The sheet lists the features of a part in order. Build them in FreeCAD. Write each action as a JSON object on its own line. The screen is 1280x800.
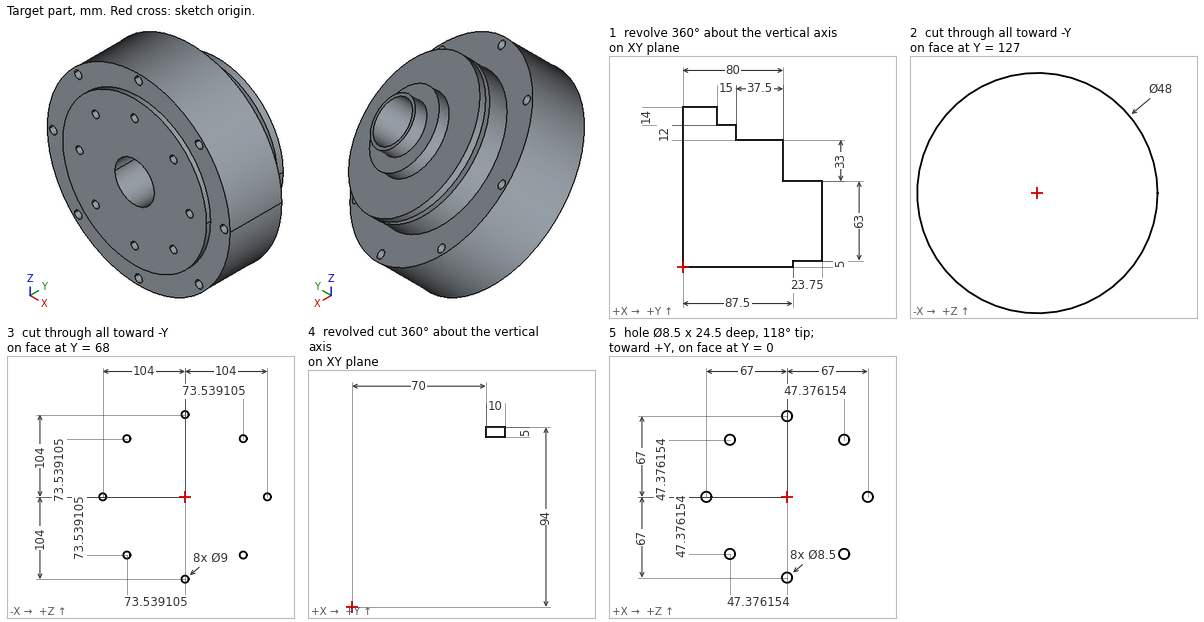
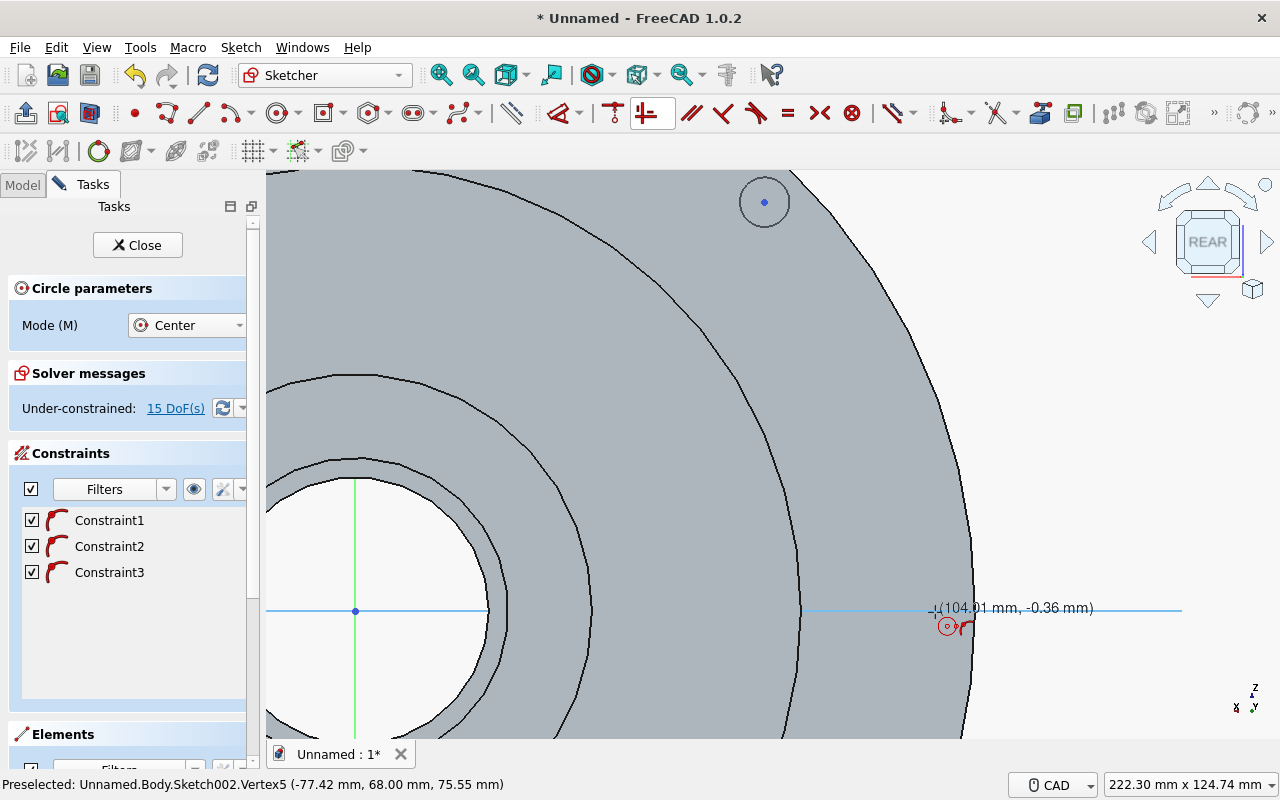
{"action": "left_click", "coordinate": [935, 611]}
{"action": "left_click", "coordinate": [952, 593]}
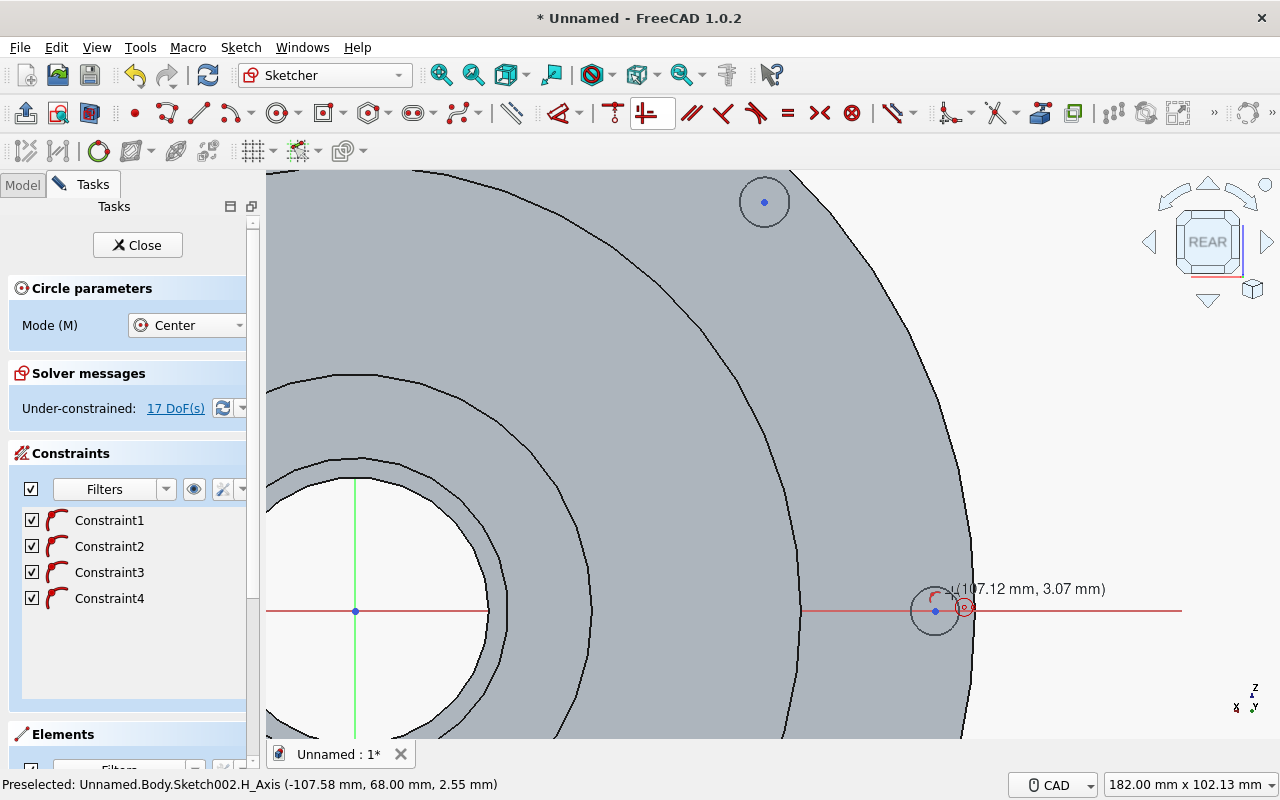
{"action": "scroll", "coordinate": [855, 387], "scroll_direction": "down", "scroll_amount": 6}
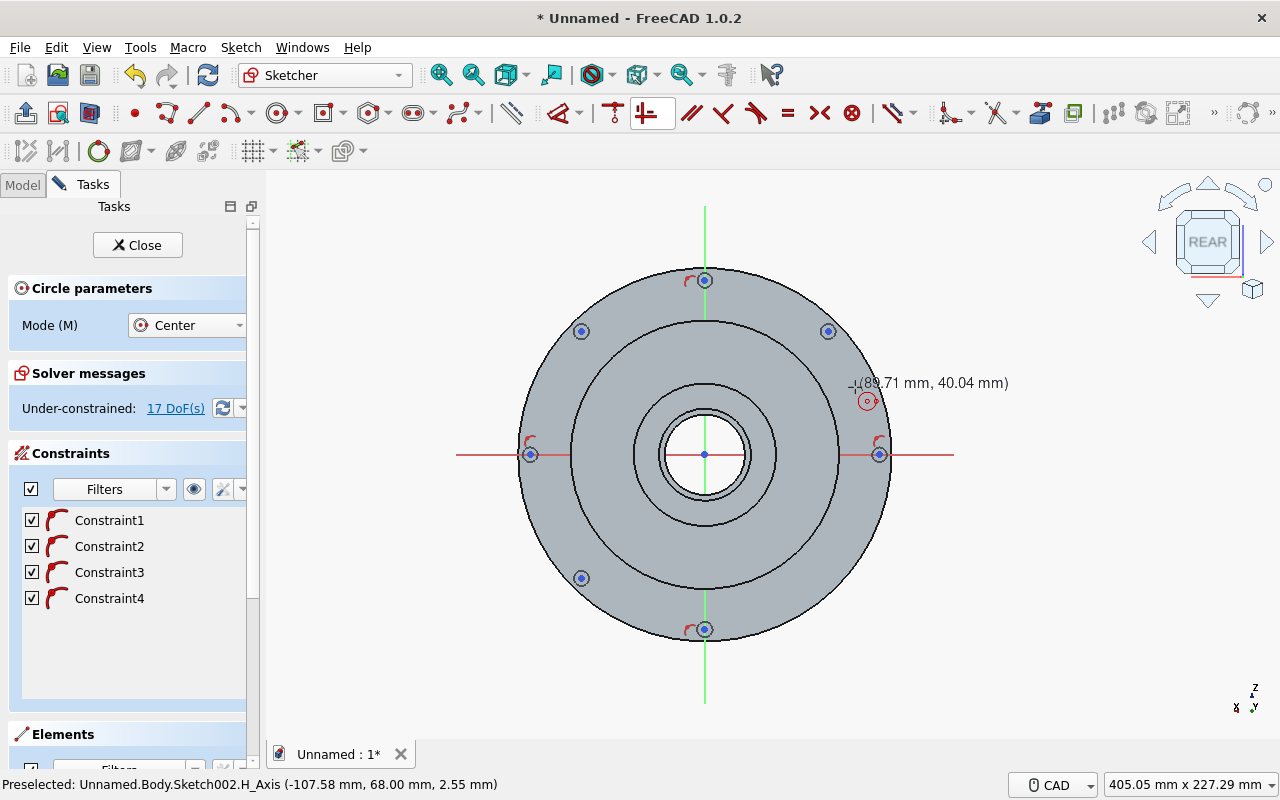
{"action": "scroll", "coordinate": [828, 578], "scroll_direction": "up", "scroll_amount": 6}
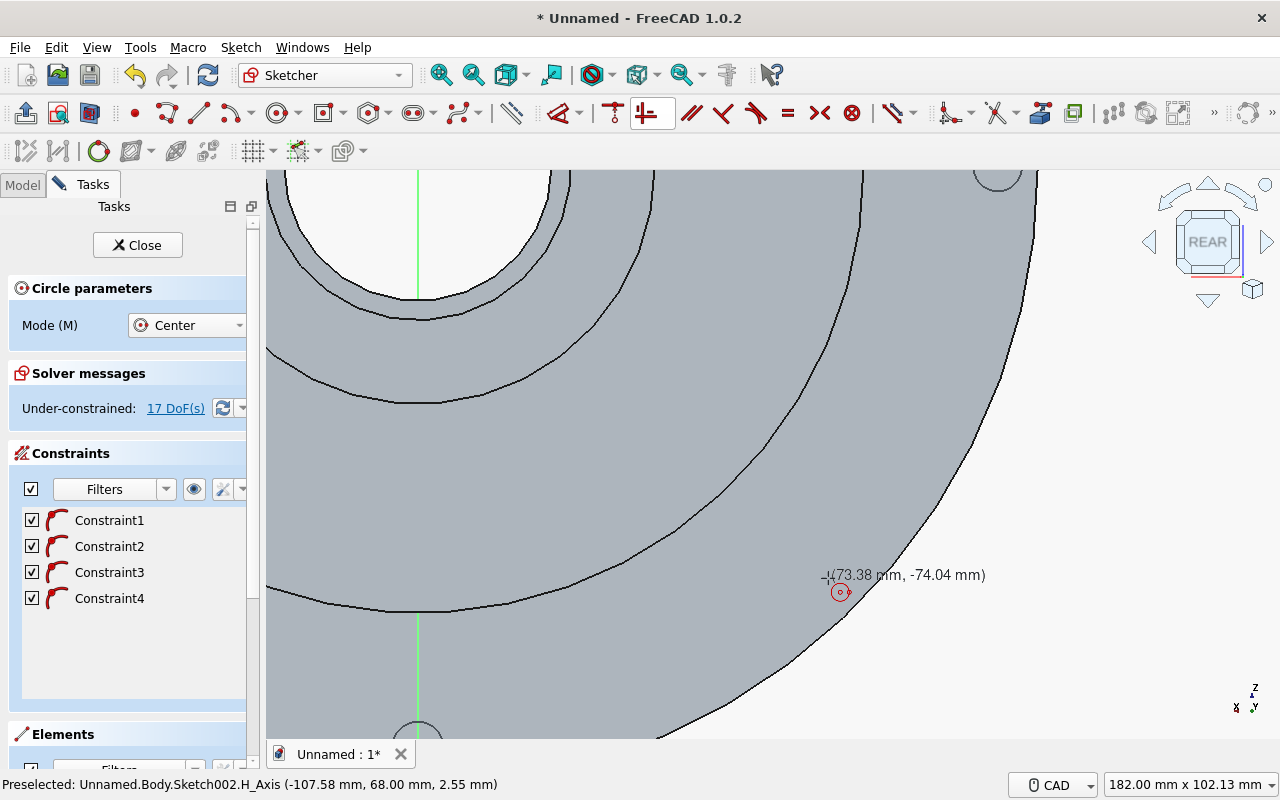
{"action": "left_click", "coordinate": [828, 577]}
{"action": "left_click", "coordinate": [845, 559]}
{"action": "key", "text": "Escape"}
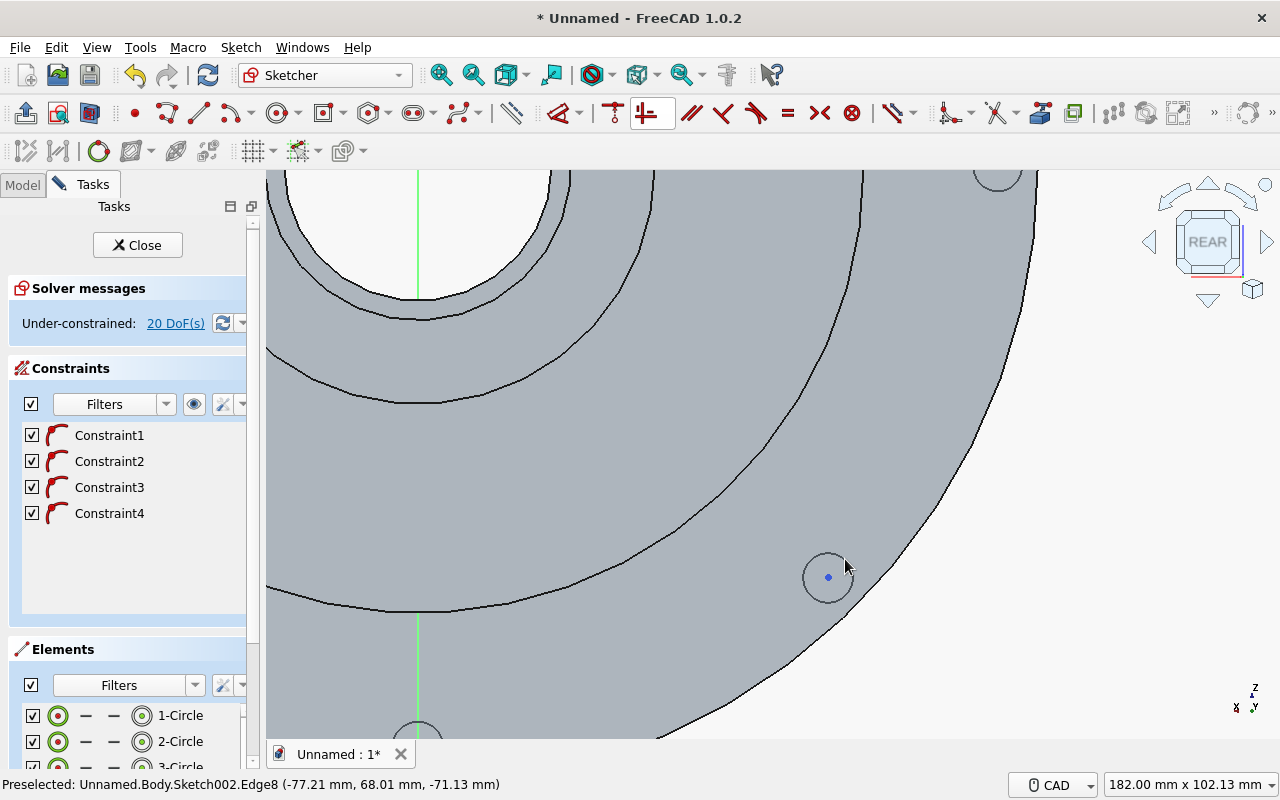
{"action": "scroll", "coordinate": [828, 578], "scroll_direction": "down", "scroll_amount": 6}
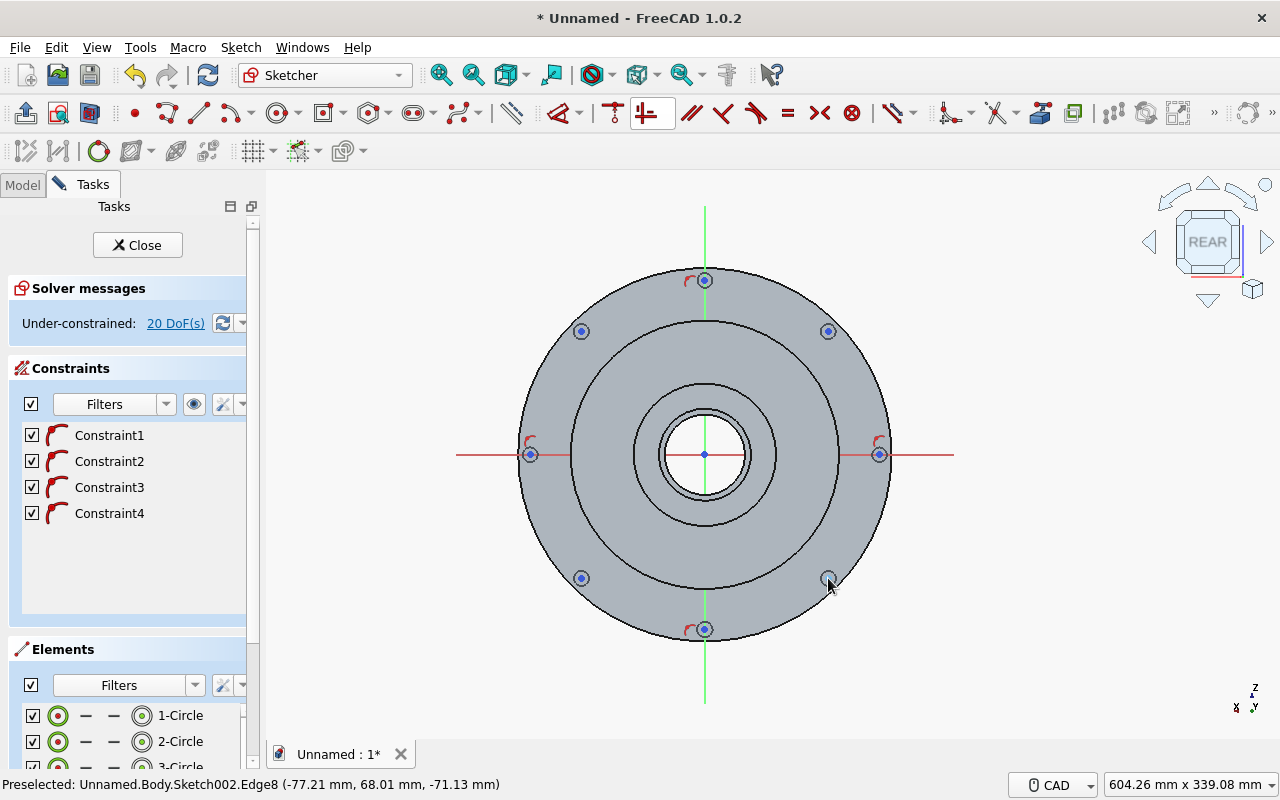
{"action": "scroll", "coordinate": [710, 624], "scroll_direction": "up", "scroll_amount": 5}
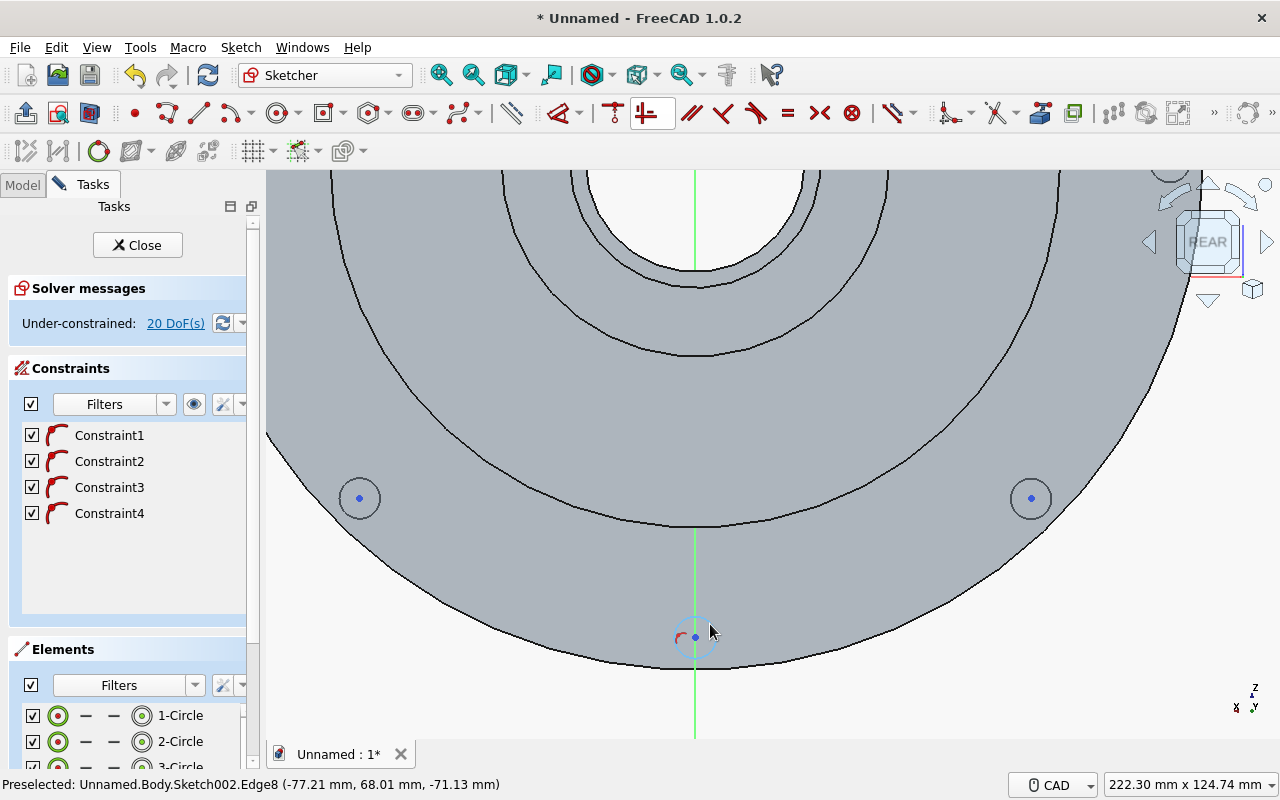
{"action": "left_click", "coordinate": [710, 623]}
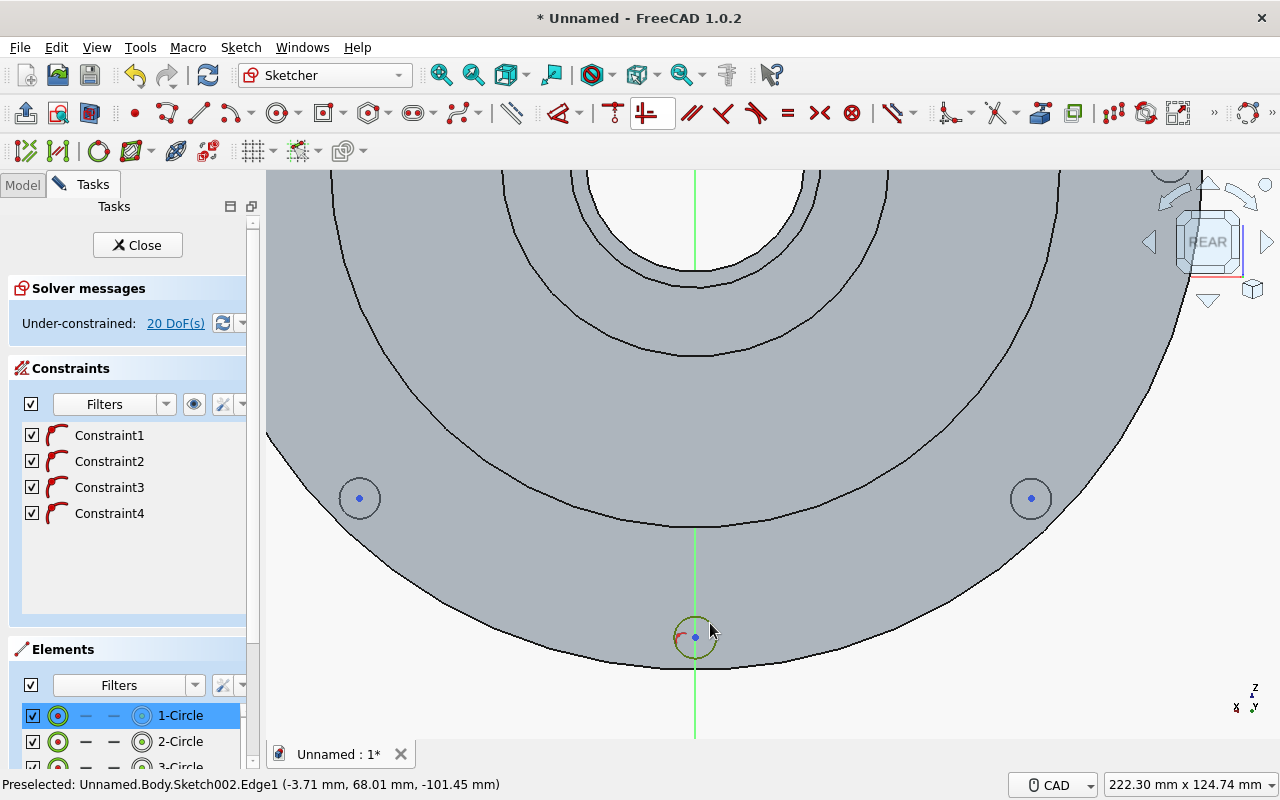
{"action": "left_click", "coordinate": [374, 484]}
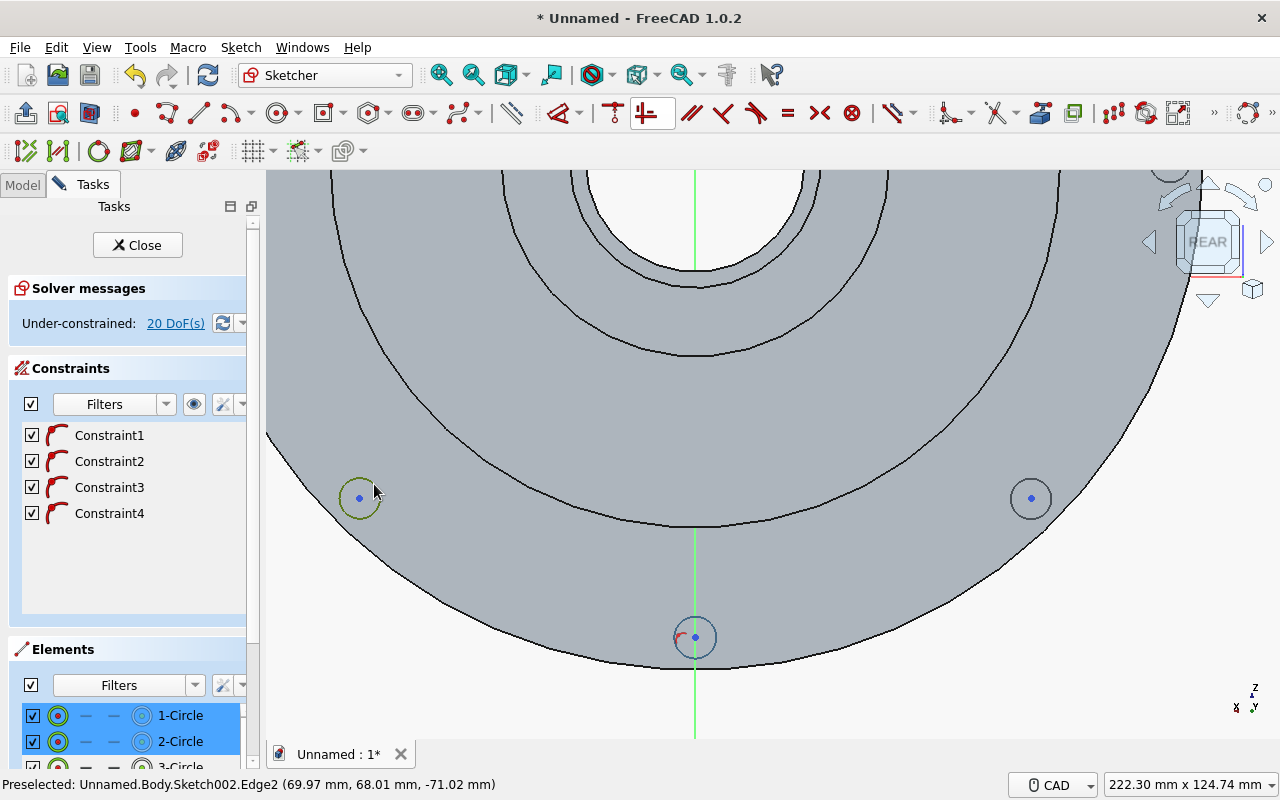
{"action": "scroll", "coordinate": [710, 624], "scroll_direction": "down", "scroll_amount": 5}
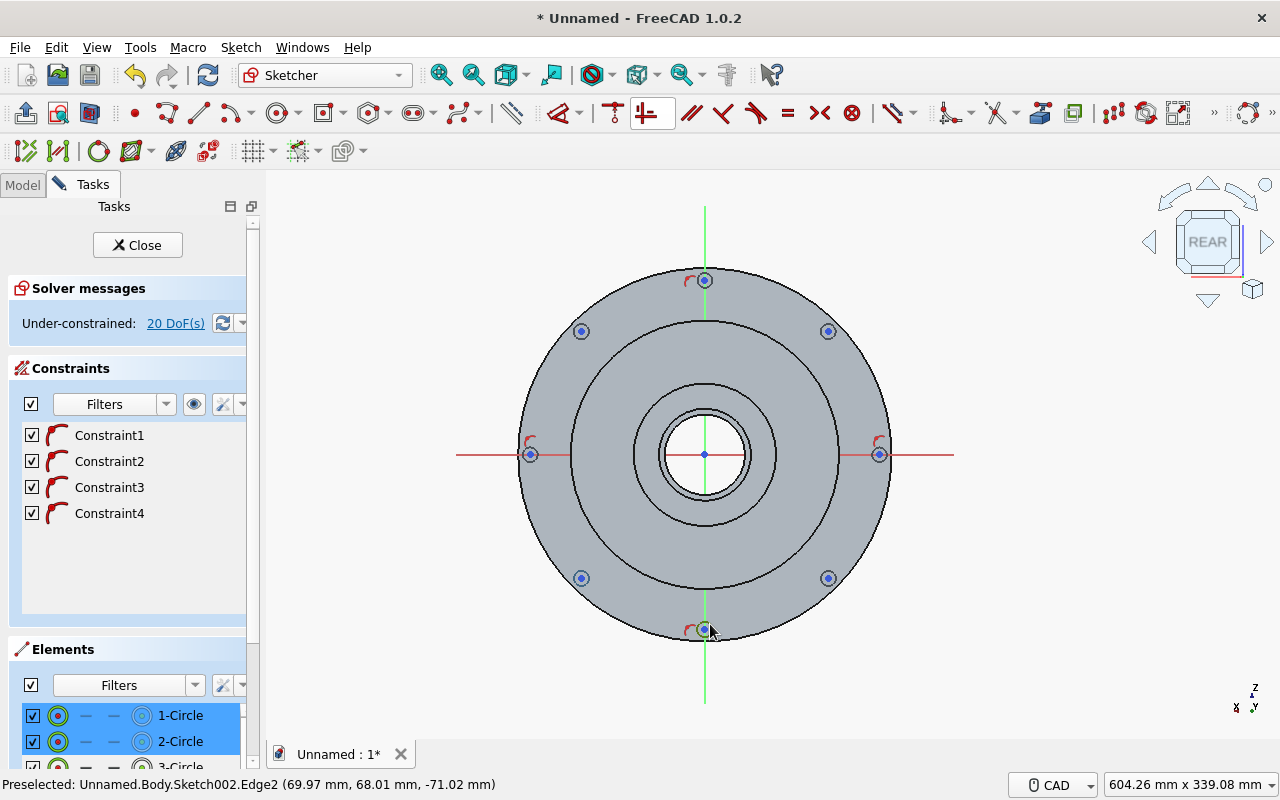
{"action": "scroll", "coordinate": [535, 450], "scroll_direction": "up", "scroll_amount": 5}